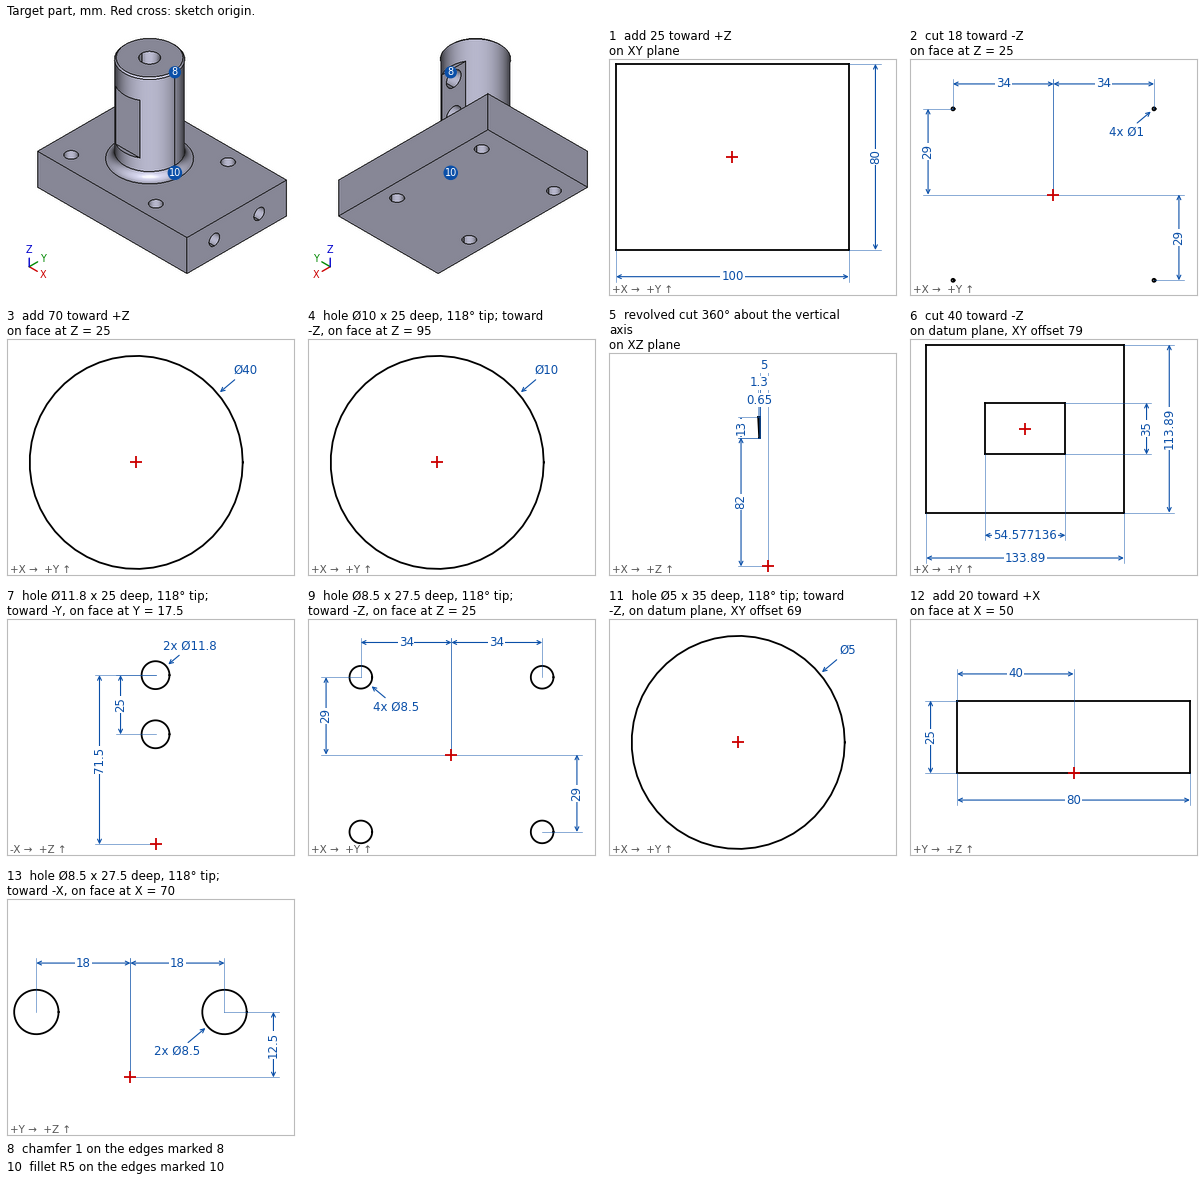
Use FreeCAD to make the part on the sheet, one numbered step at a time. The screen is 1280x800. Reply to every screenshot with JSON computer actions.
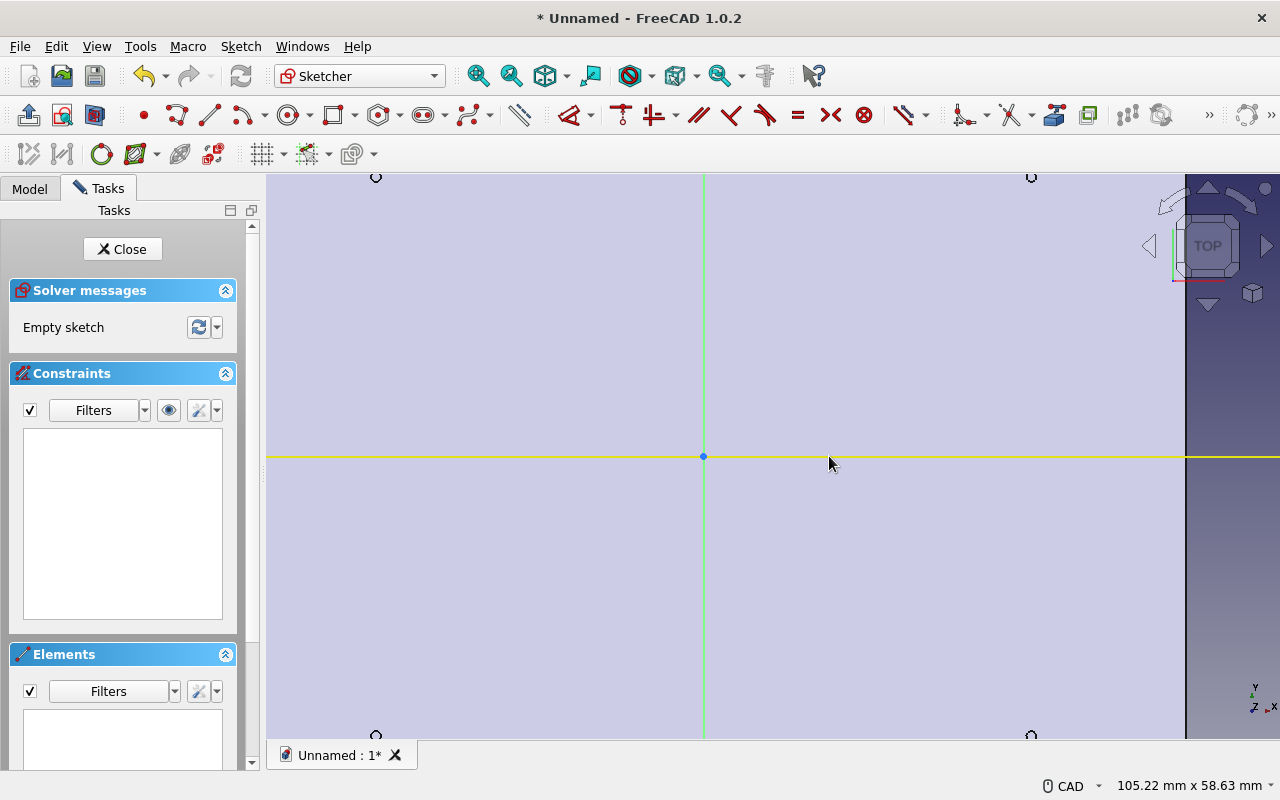
{"action": "key", "text": "g c"}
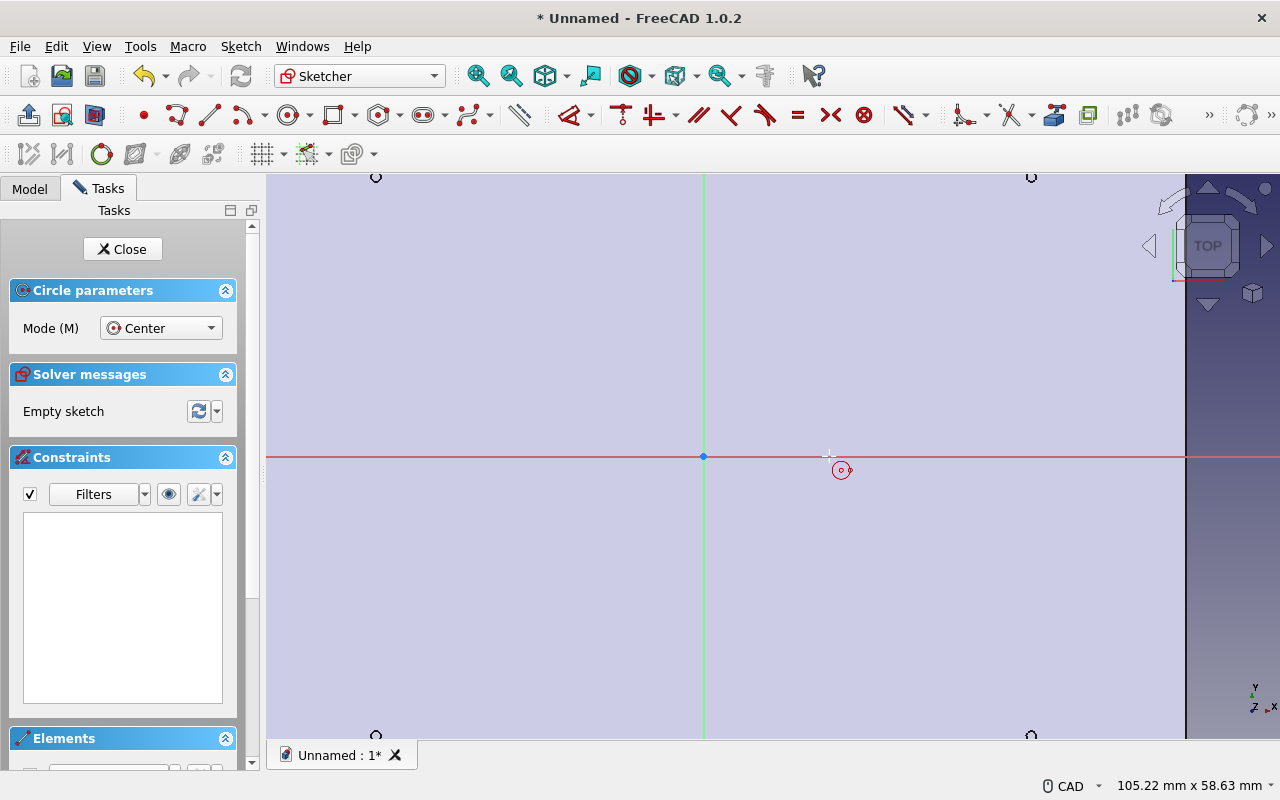
{"action": "left_click", "coordinate": [704, 456]}
{"action": "mouse_move", "coordinate": [840, 320]}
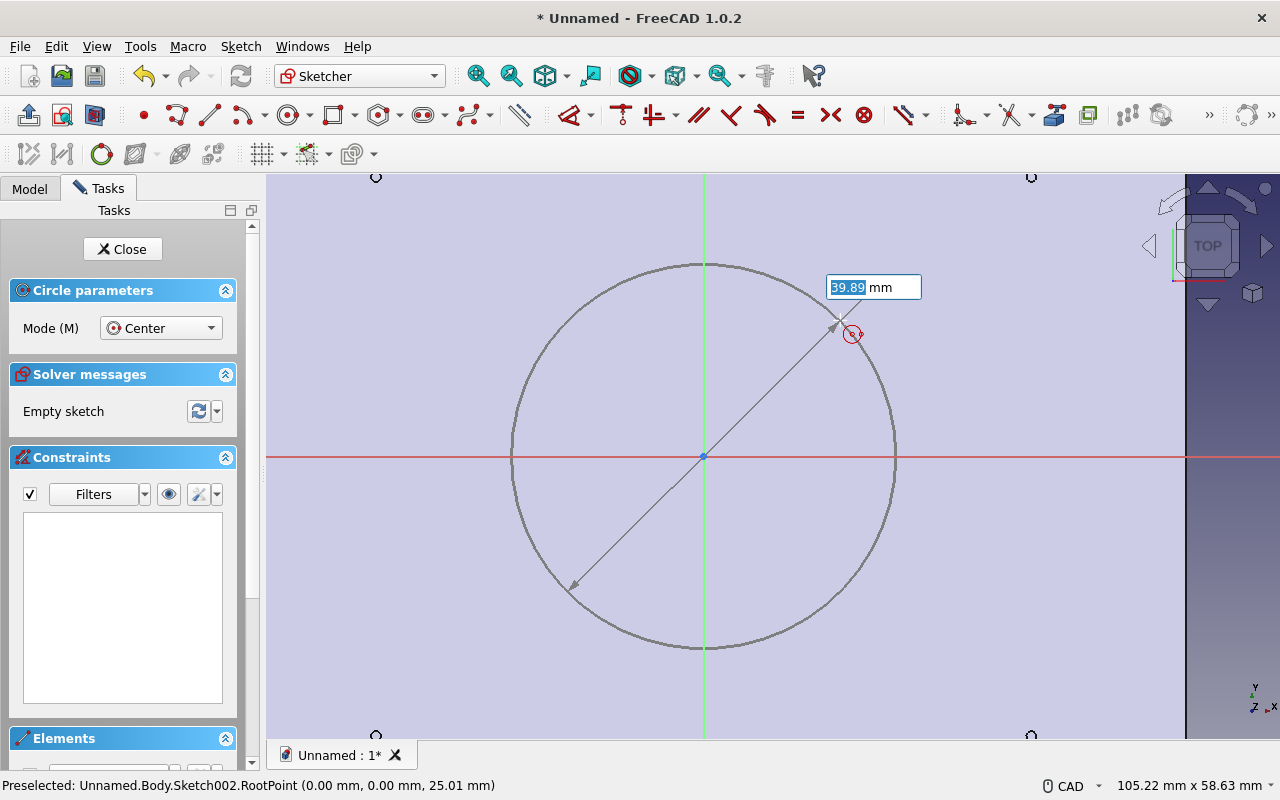
{"action": "type", "text": "40"}
{"action": "key", "text": "Return"}
{"action": "key", "text": "Escape"}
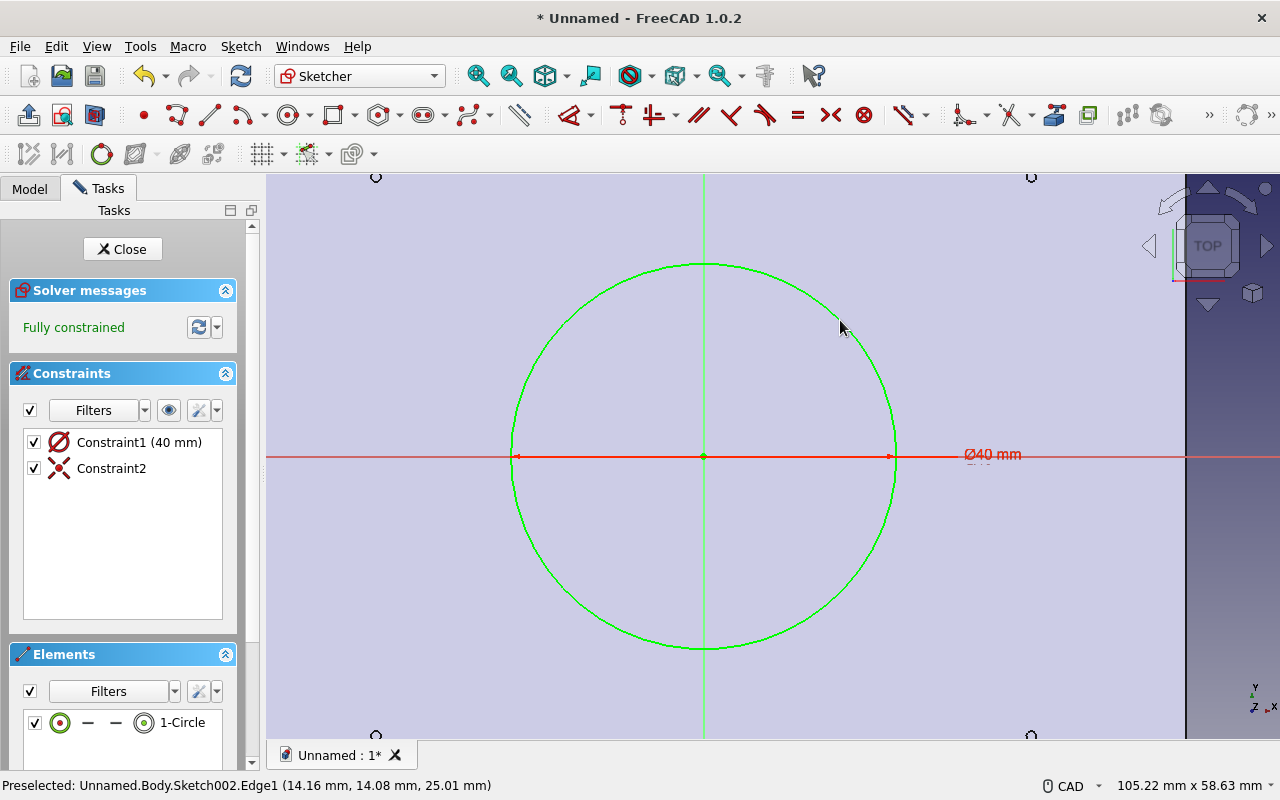
{"action": "left_click", "coordinate": [123, 249]}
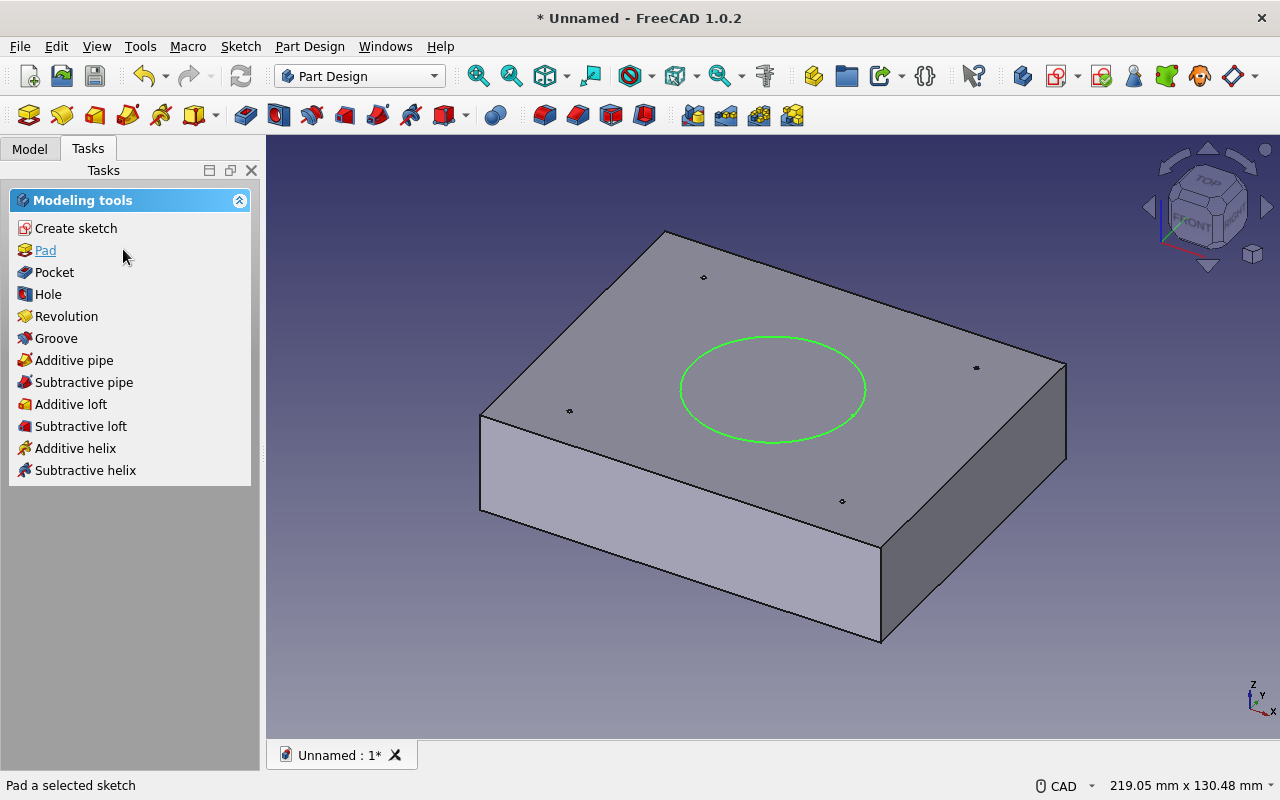
{"action": "left_click", "coordinate": [29, 116]}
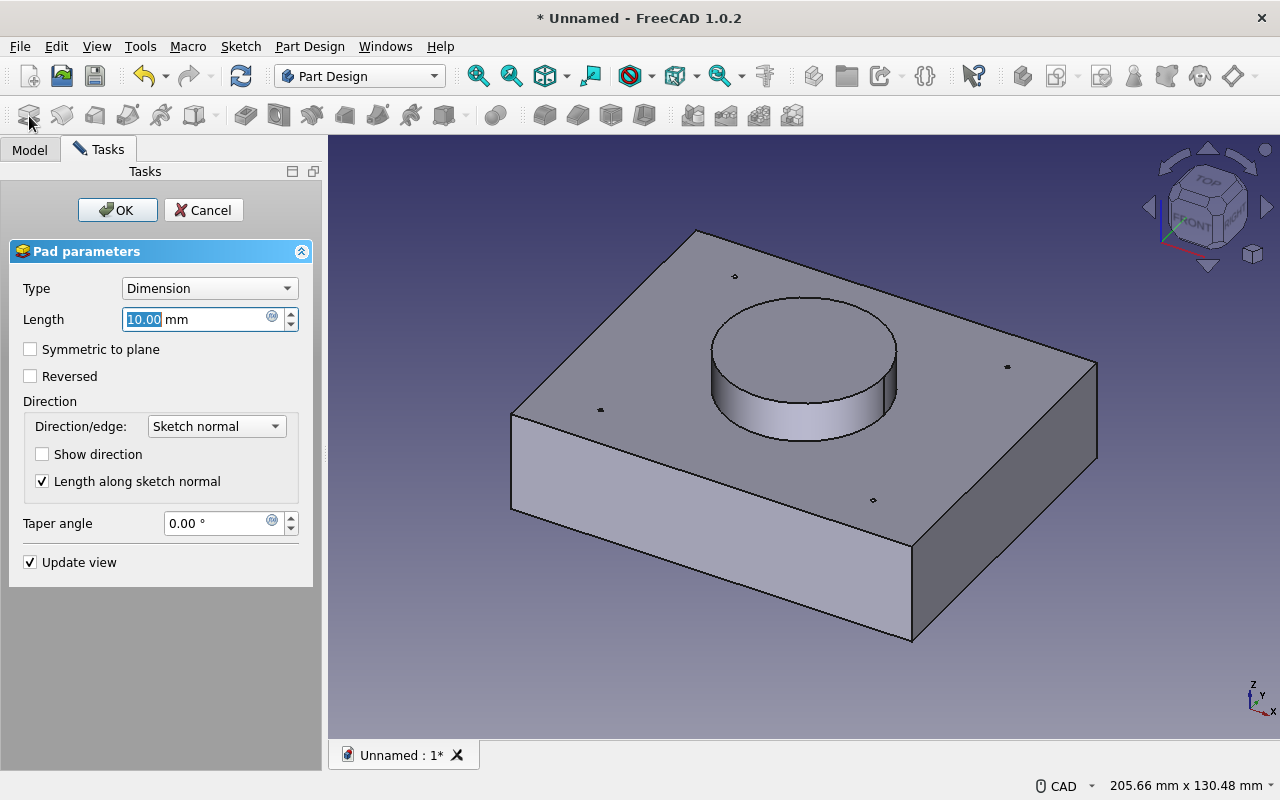
{"action": "type", "text": "70"}
{"action": "key", "text": "Tab"}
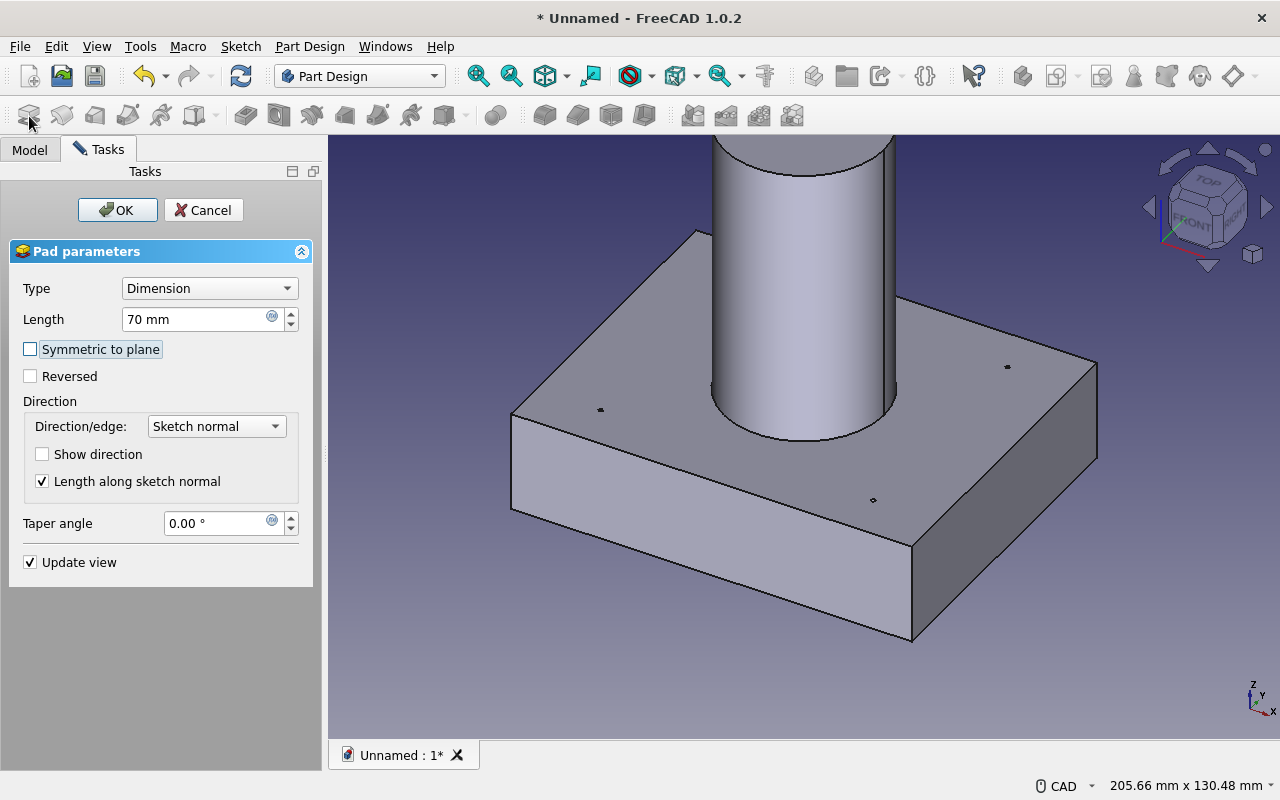
{"action": "left_click", "coordinate": [118, 210]}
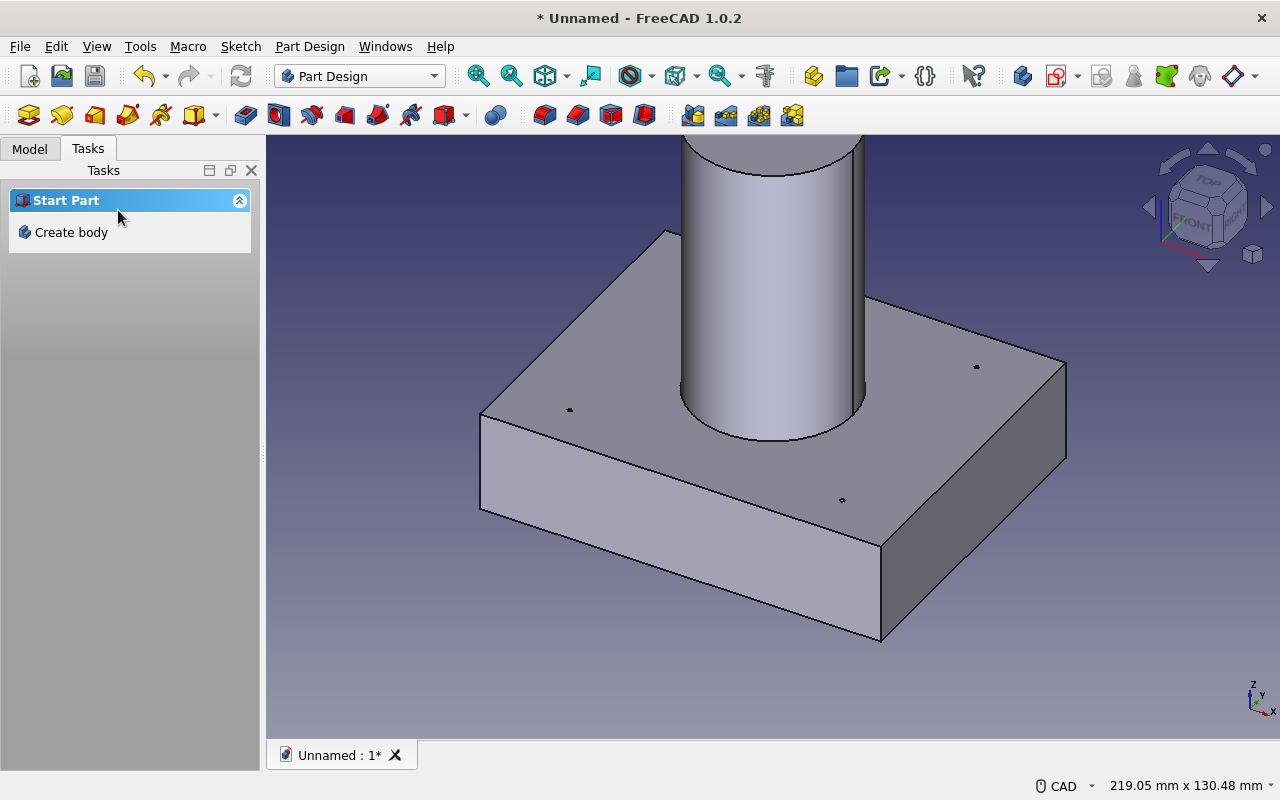
{"action": "key", "text": "v f"}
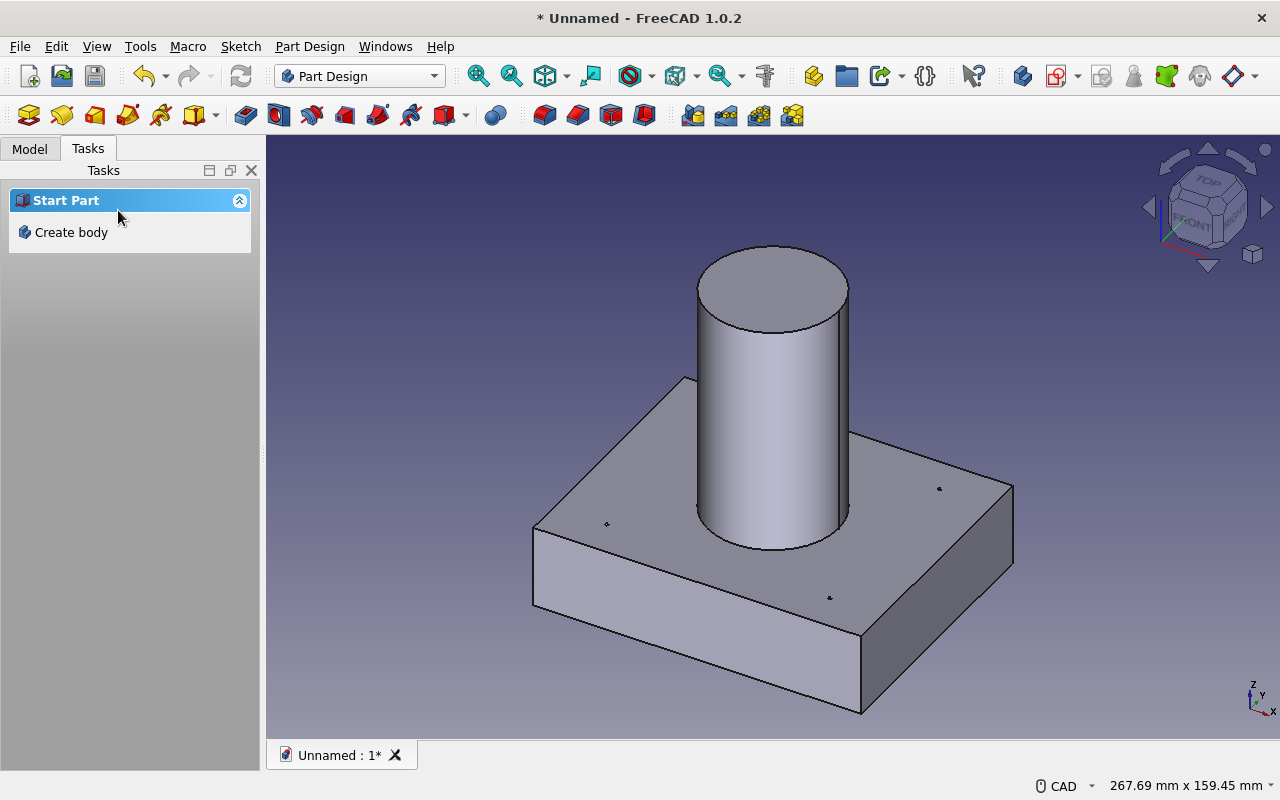
{"action": "left_click", "coordinate": [773, 289]}